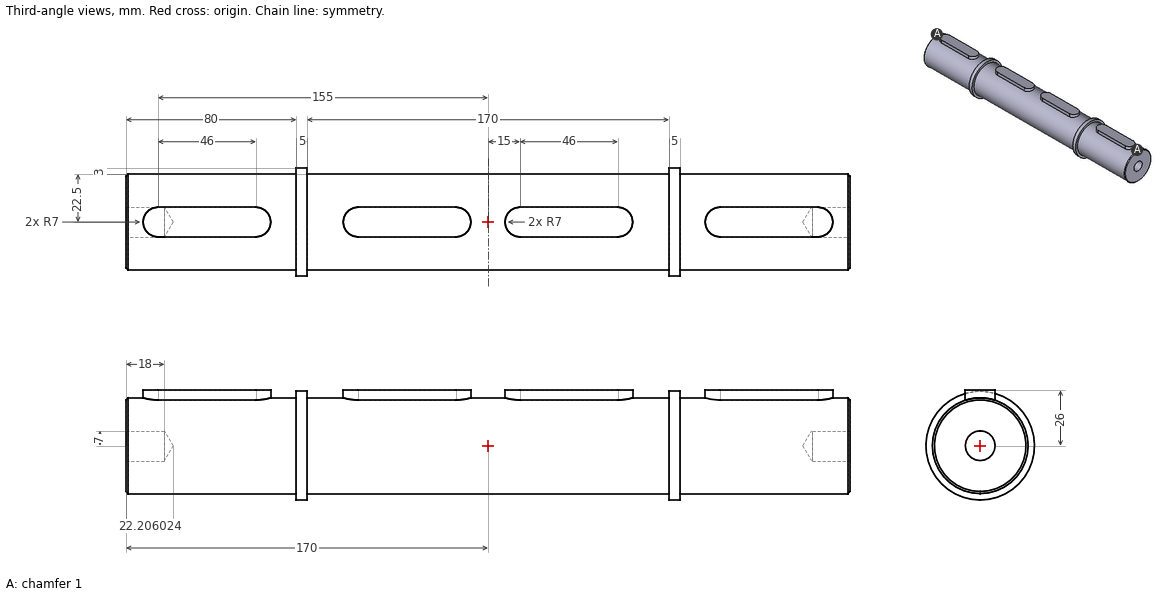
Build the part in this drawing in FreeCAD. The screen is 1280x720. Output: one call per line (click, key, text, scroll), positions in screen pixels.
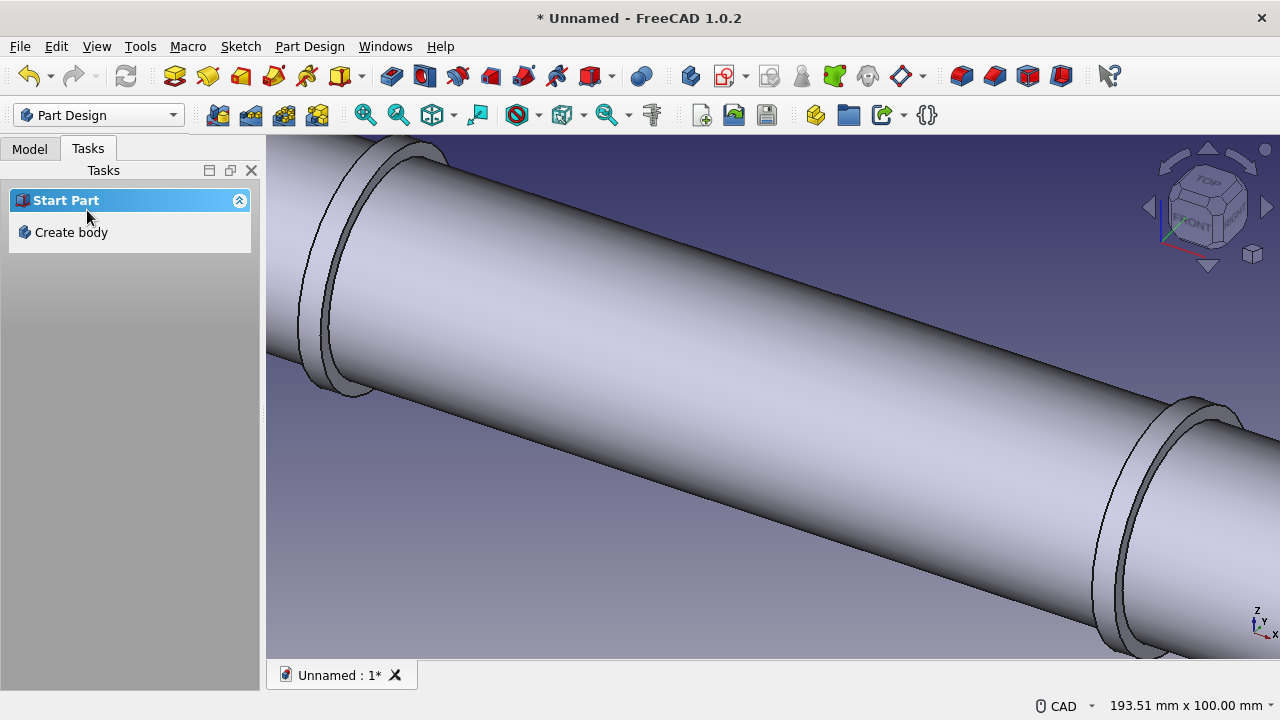
key(v)
key(f)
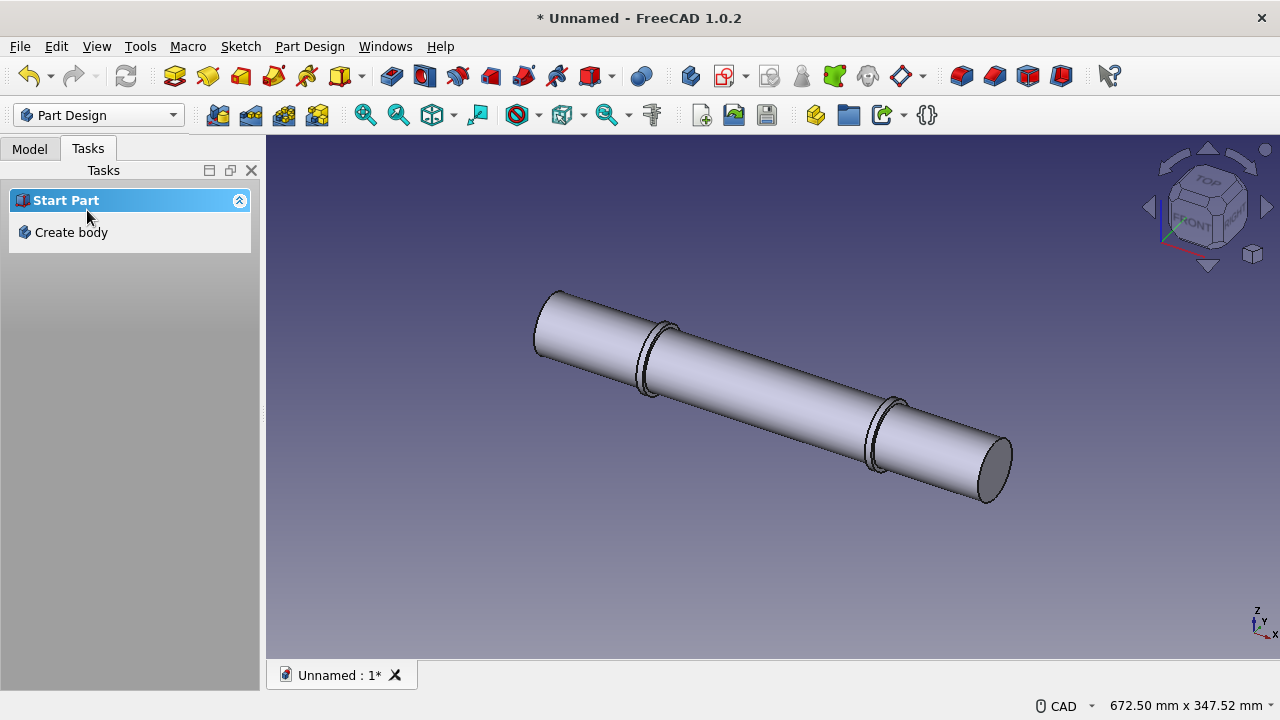
click(978, 486)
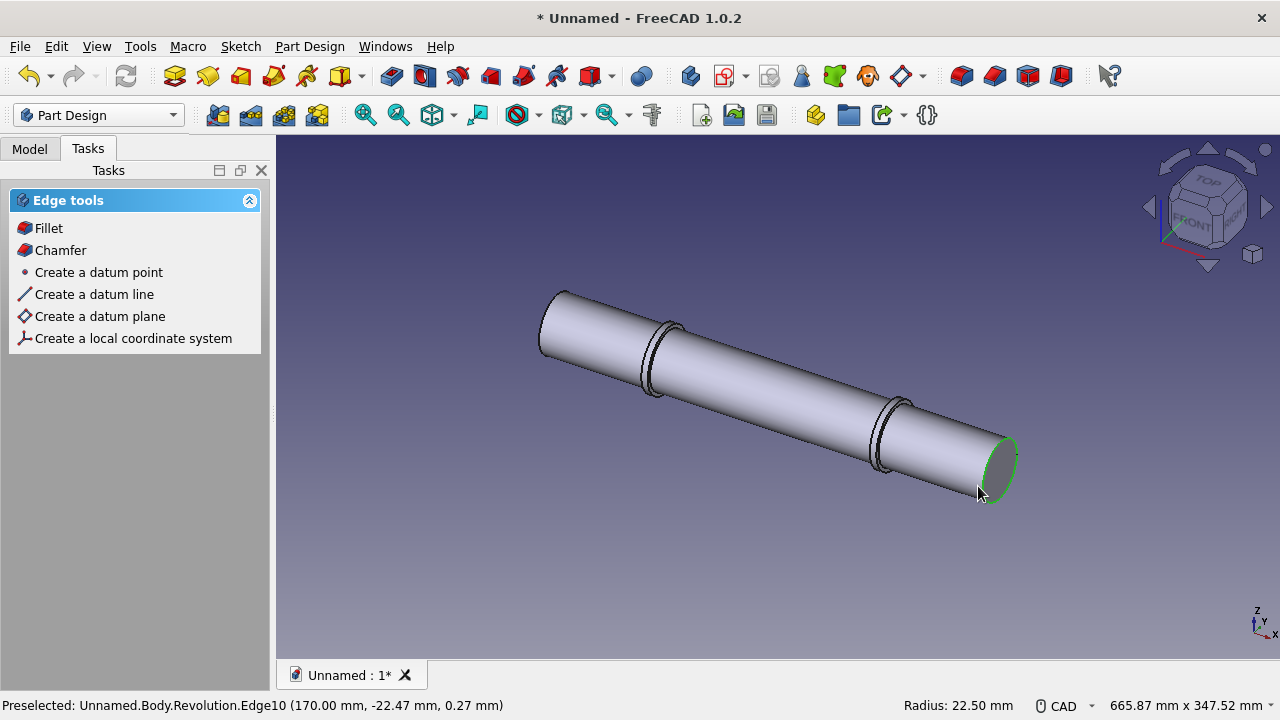
key(0)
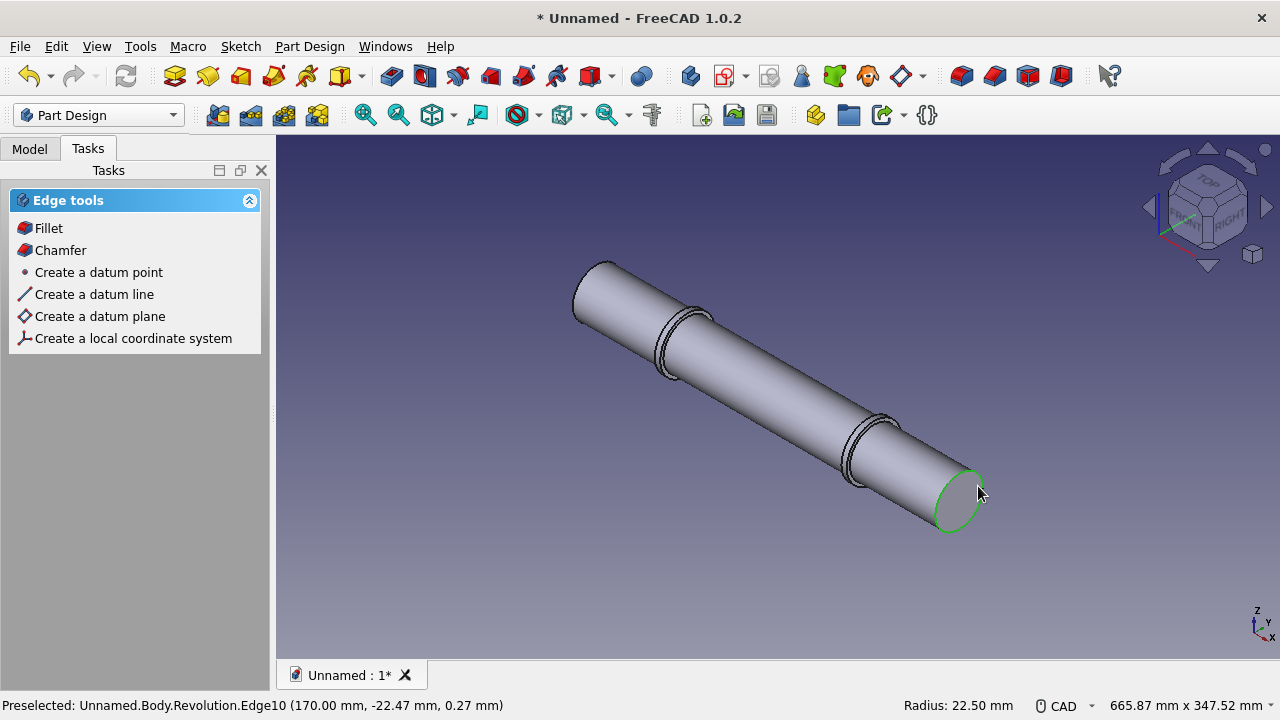
click(589, 269, ctrl)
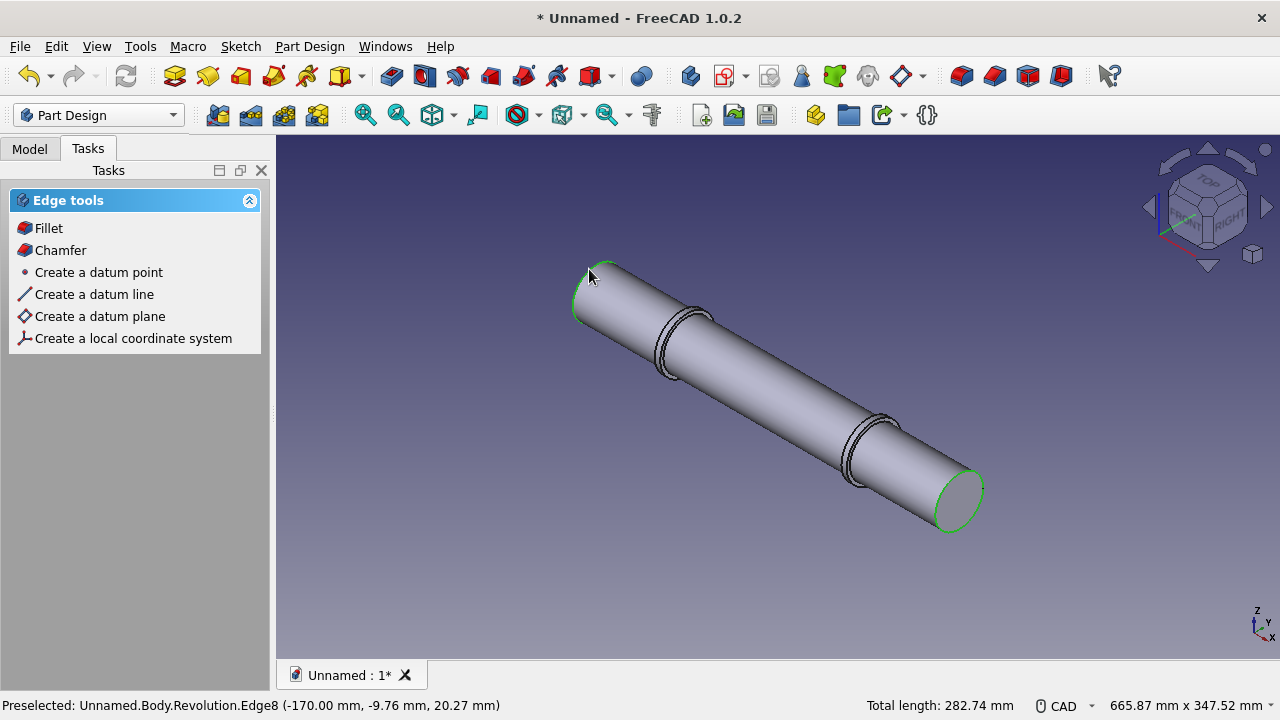
click(995, 76)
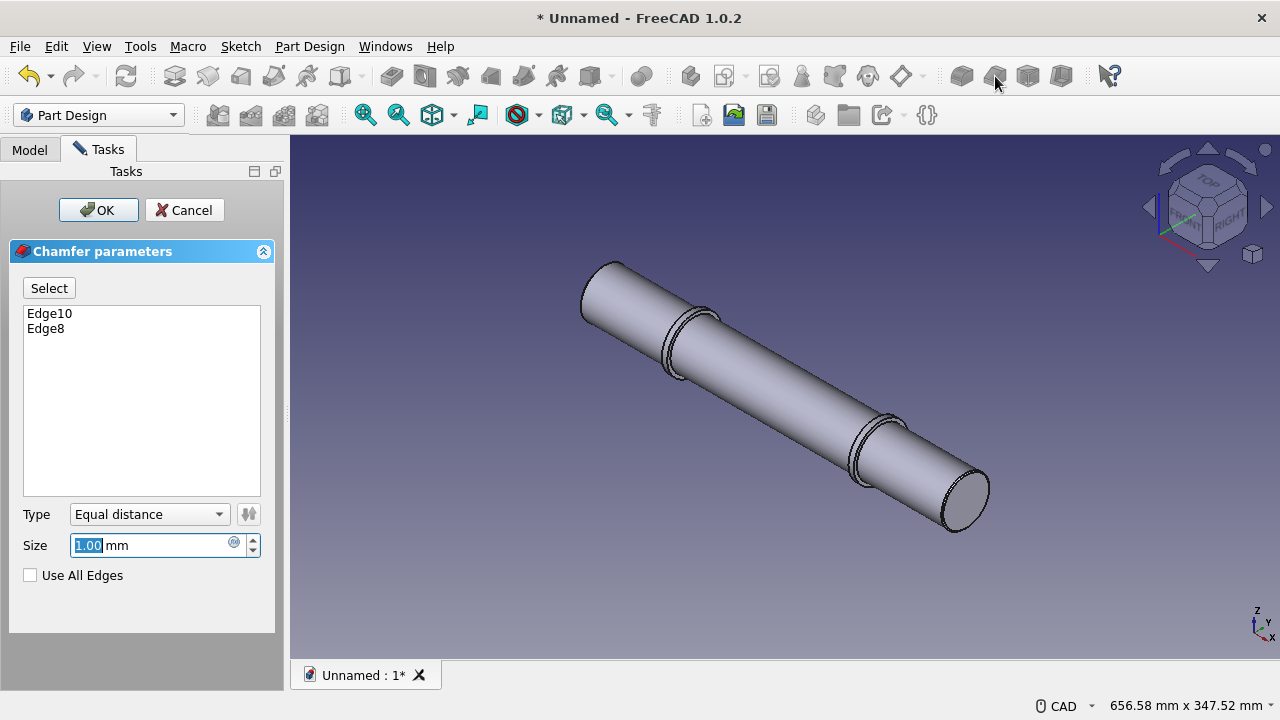
text(1)
key(Tab)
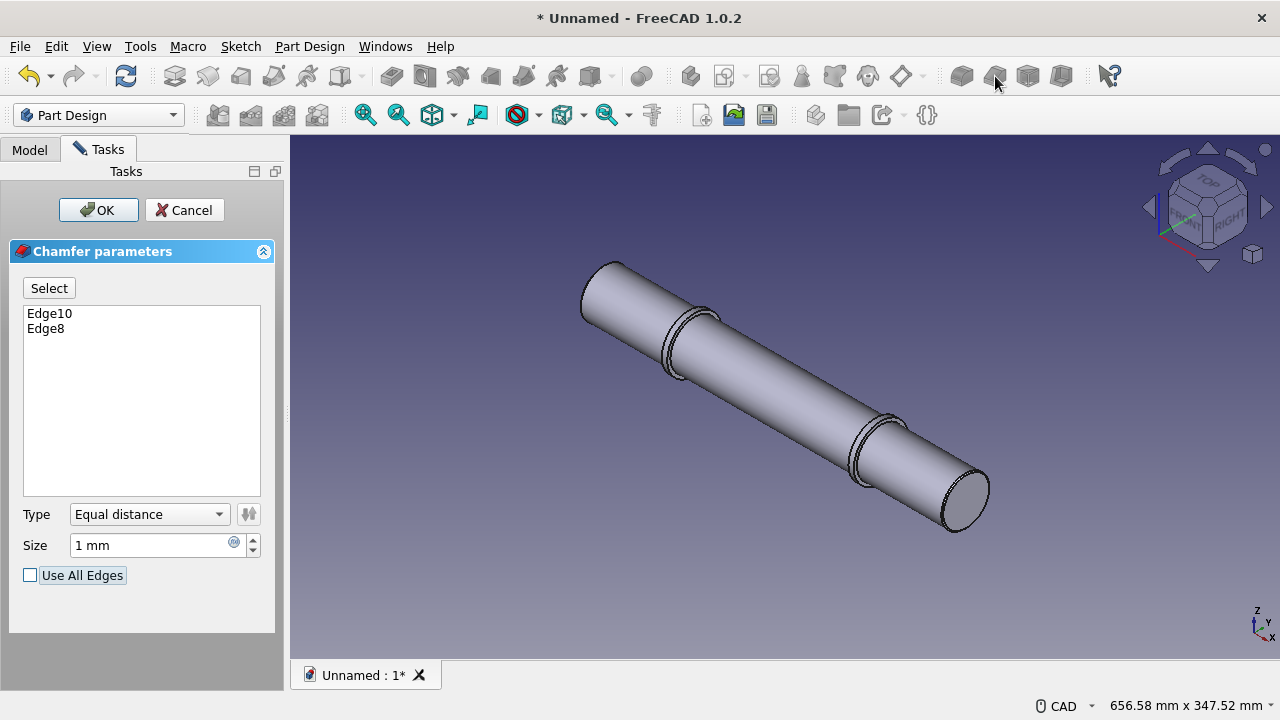
click(99, 210)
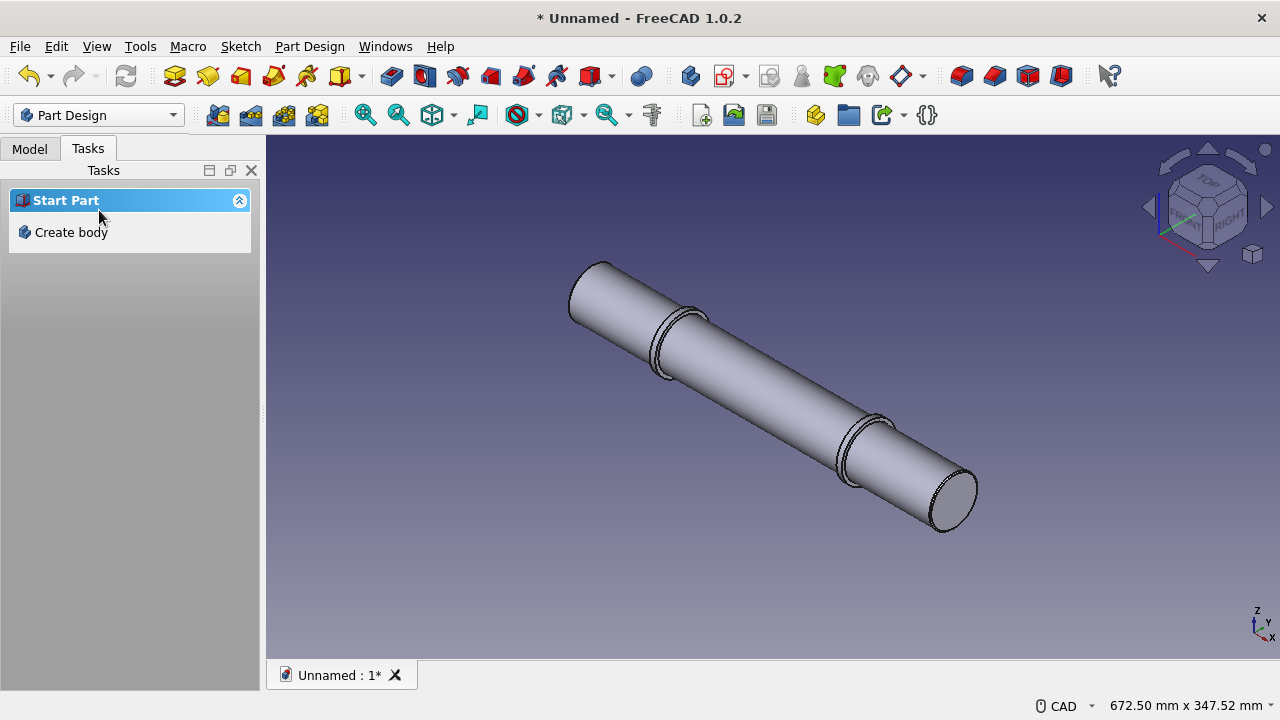
click(724, 76)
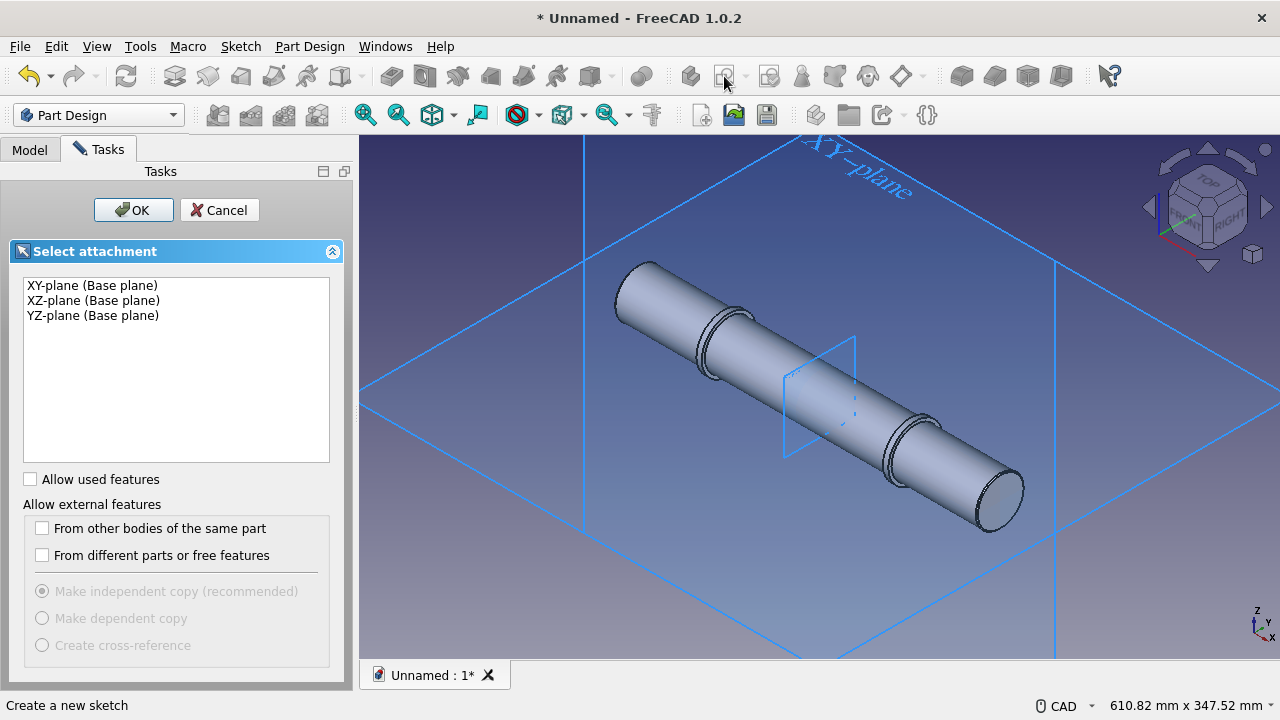
click(84, 286)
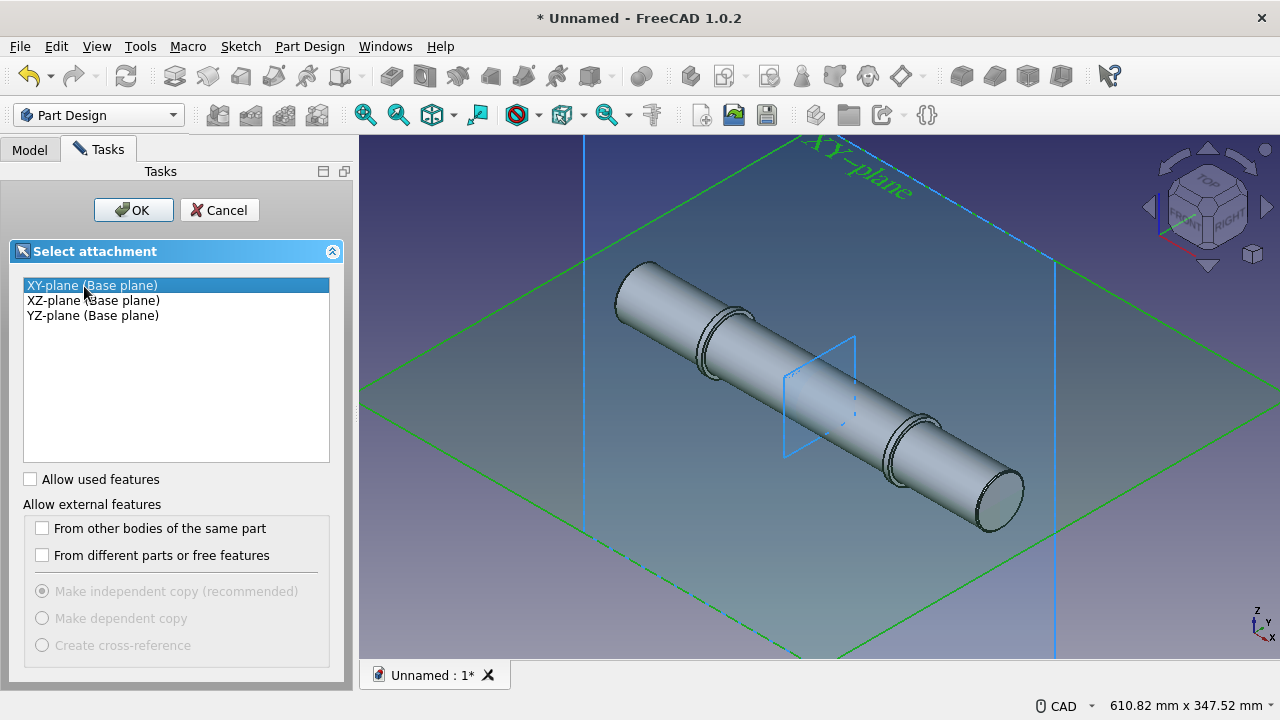
click(134, 210)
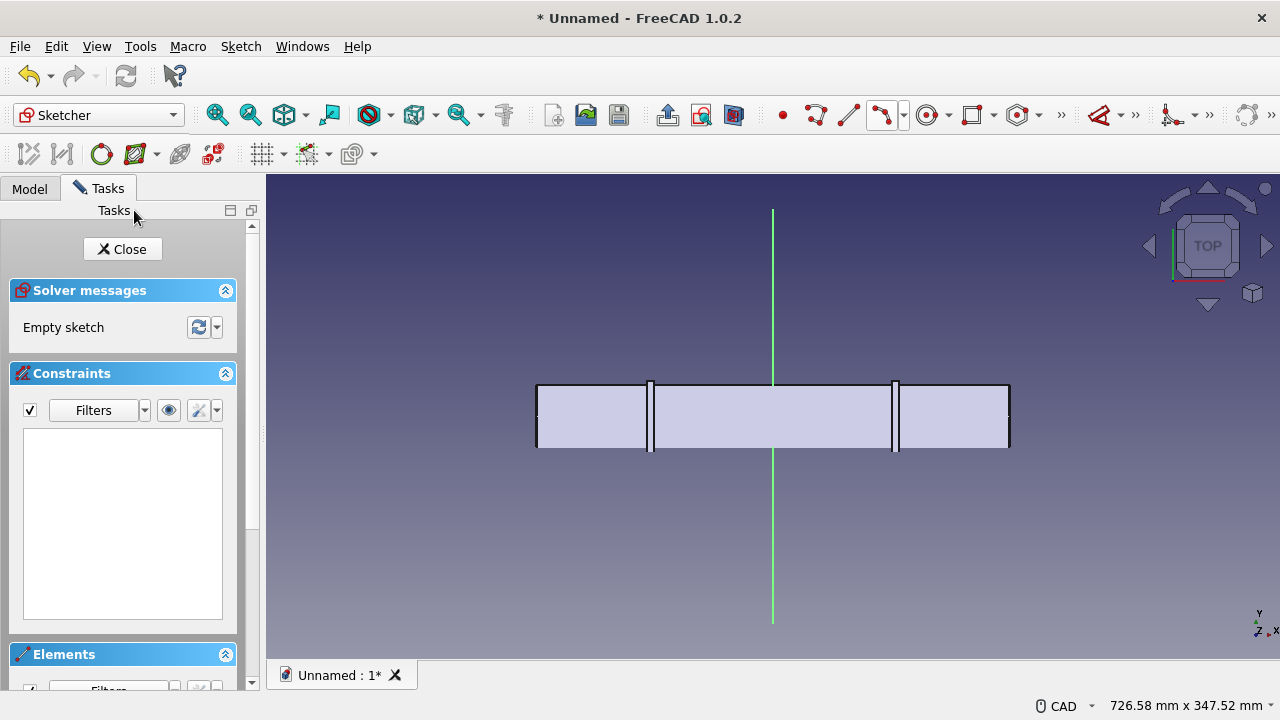
key(q)
key(s)